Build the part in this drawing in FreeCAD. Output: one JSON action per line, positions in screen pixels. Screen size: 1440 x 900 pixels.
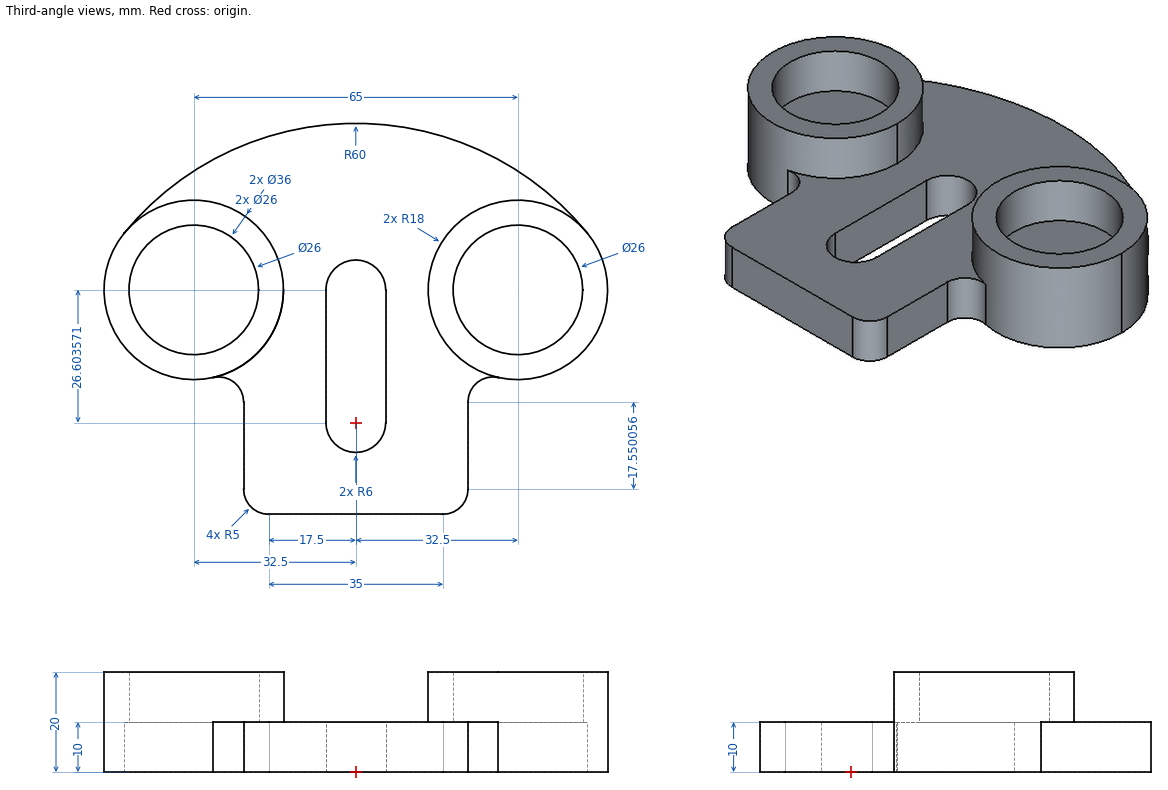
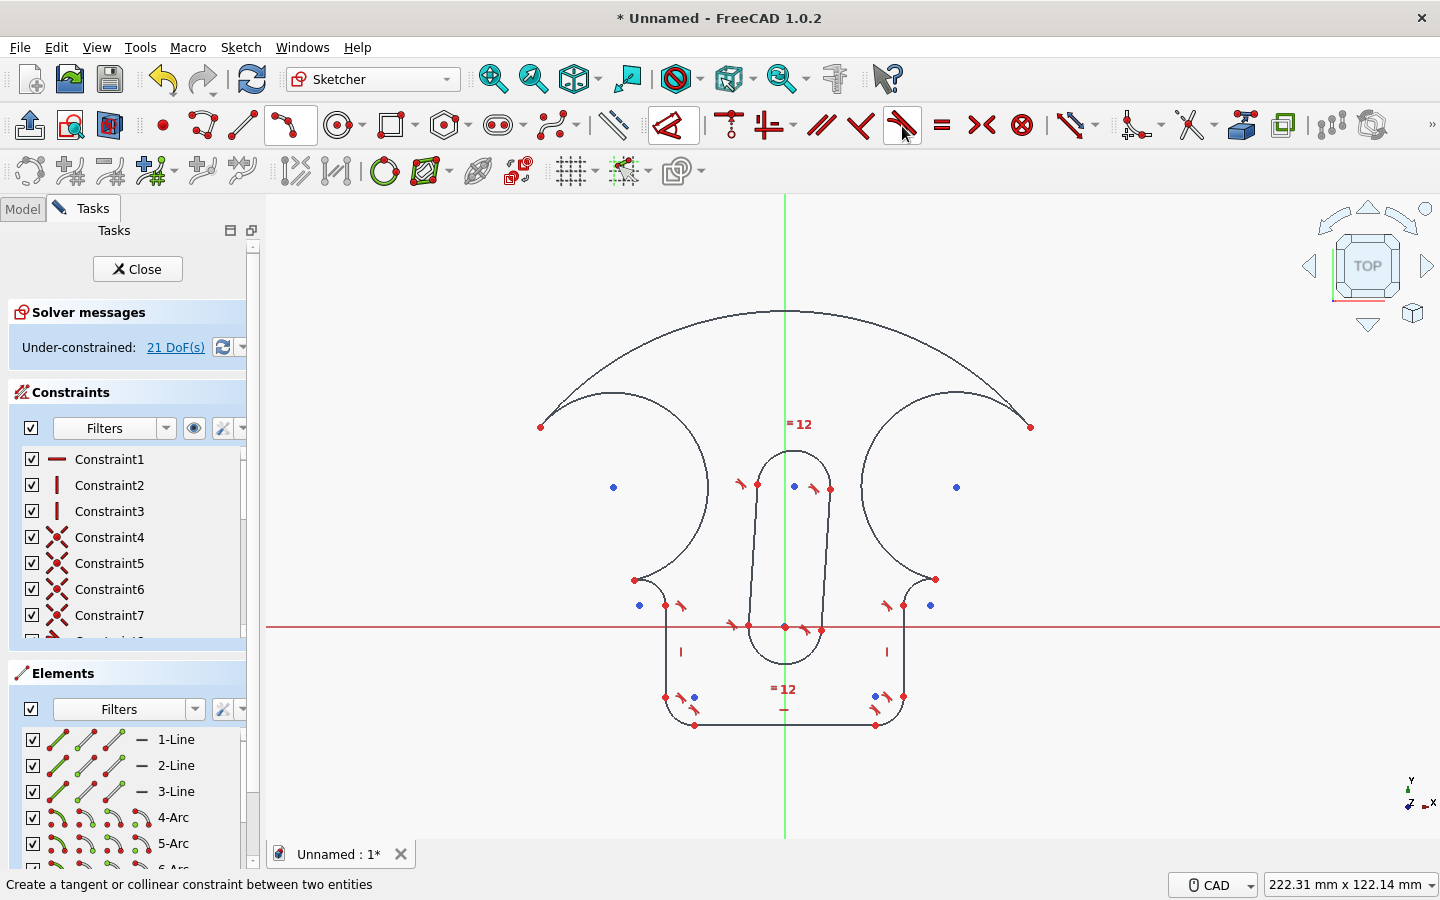
{"action": "left_click", "coordinate": [908, 592]}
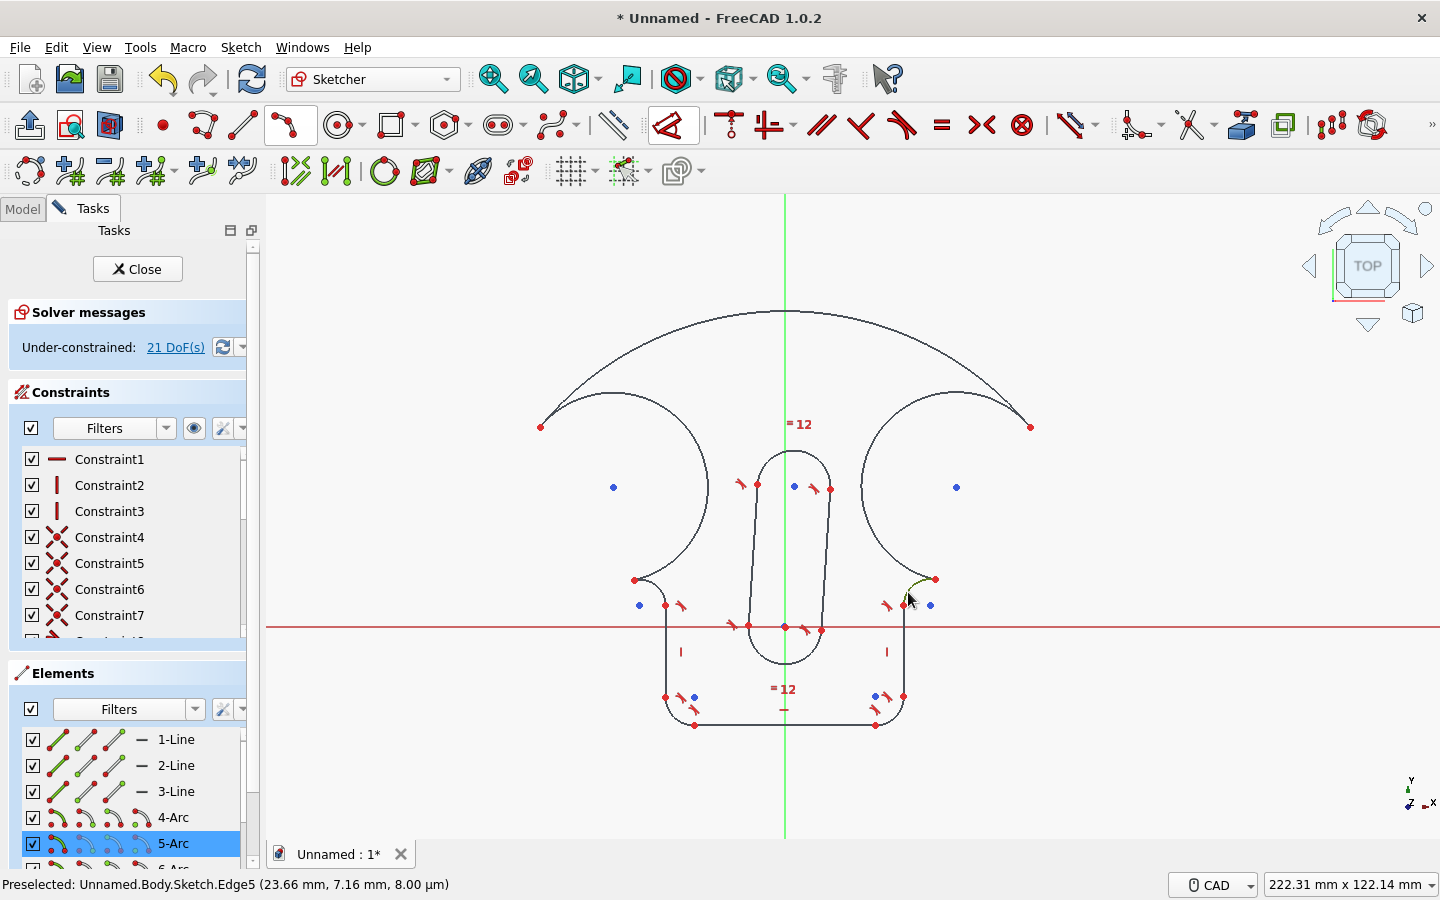
{"action": "left_click", "coordinate": [932, 395]}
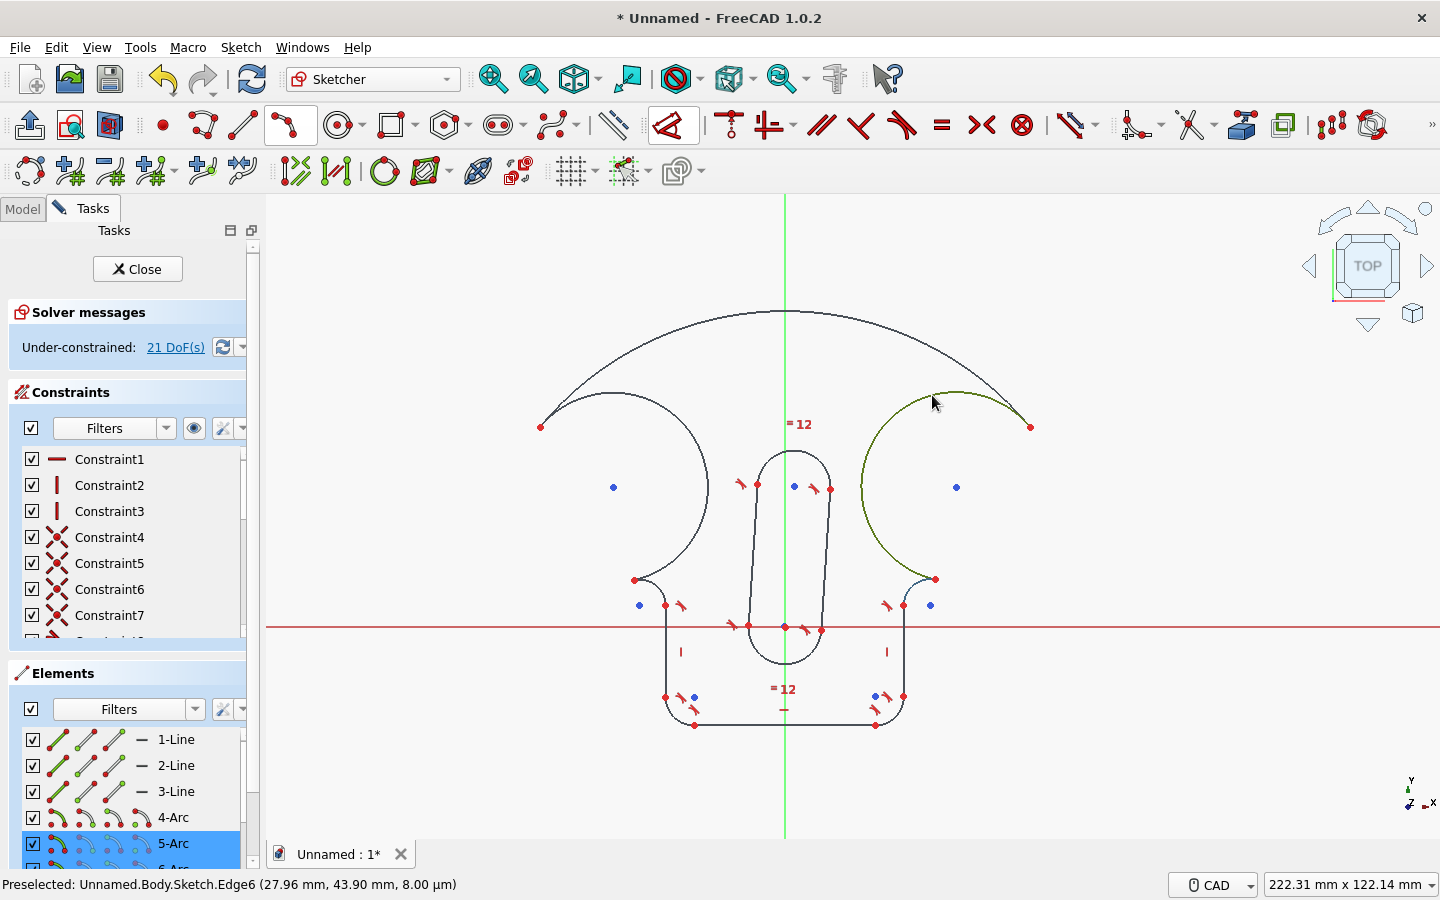
{"action": "left_click", "coordinate": [902, 126]}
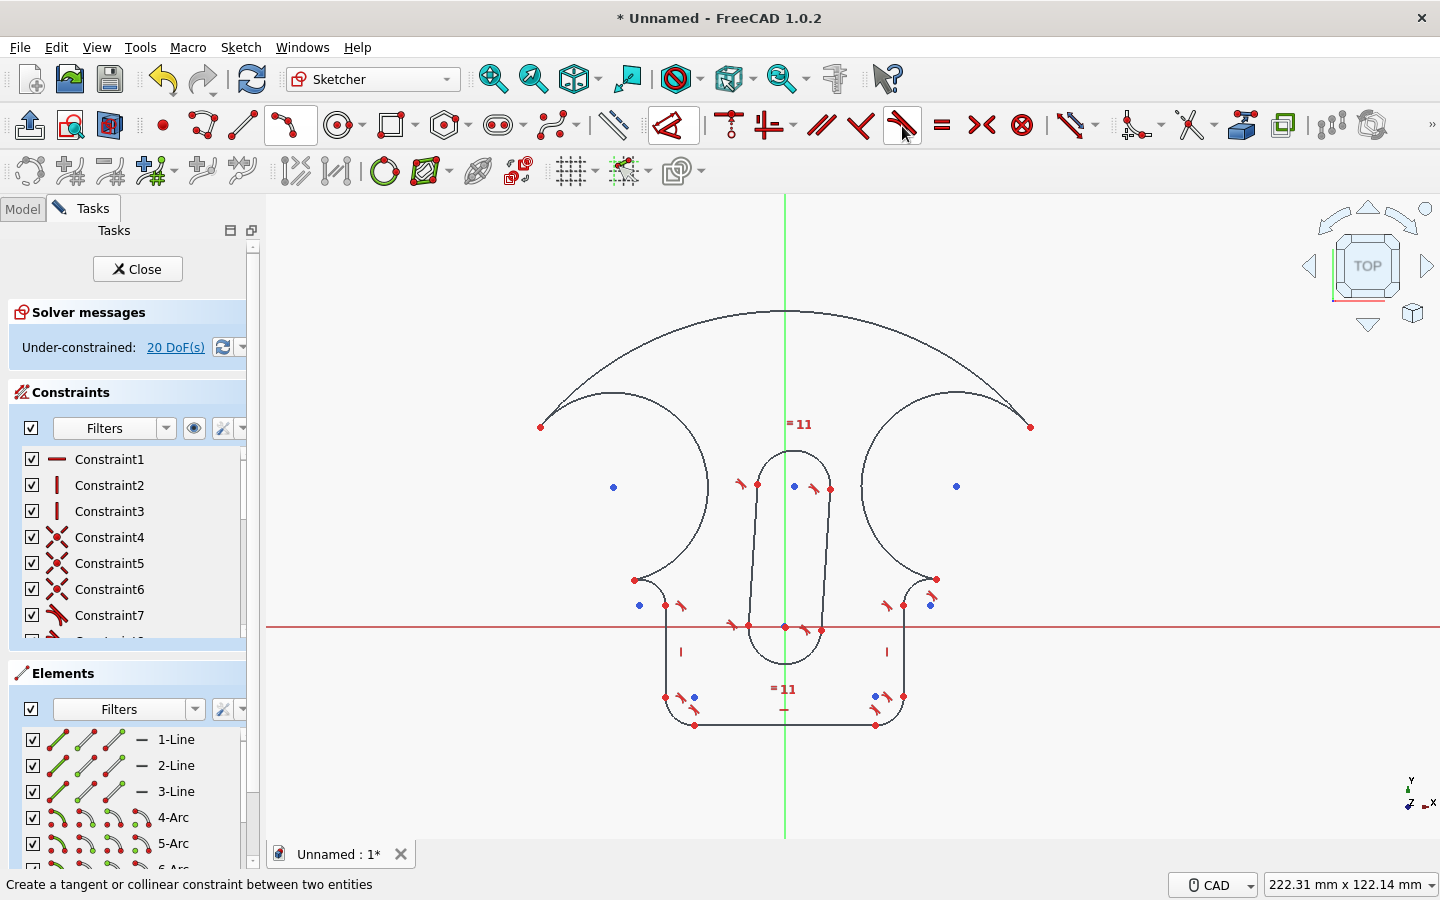
{"action": "left_click", "coordinate": [932, 395]}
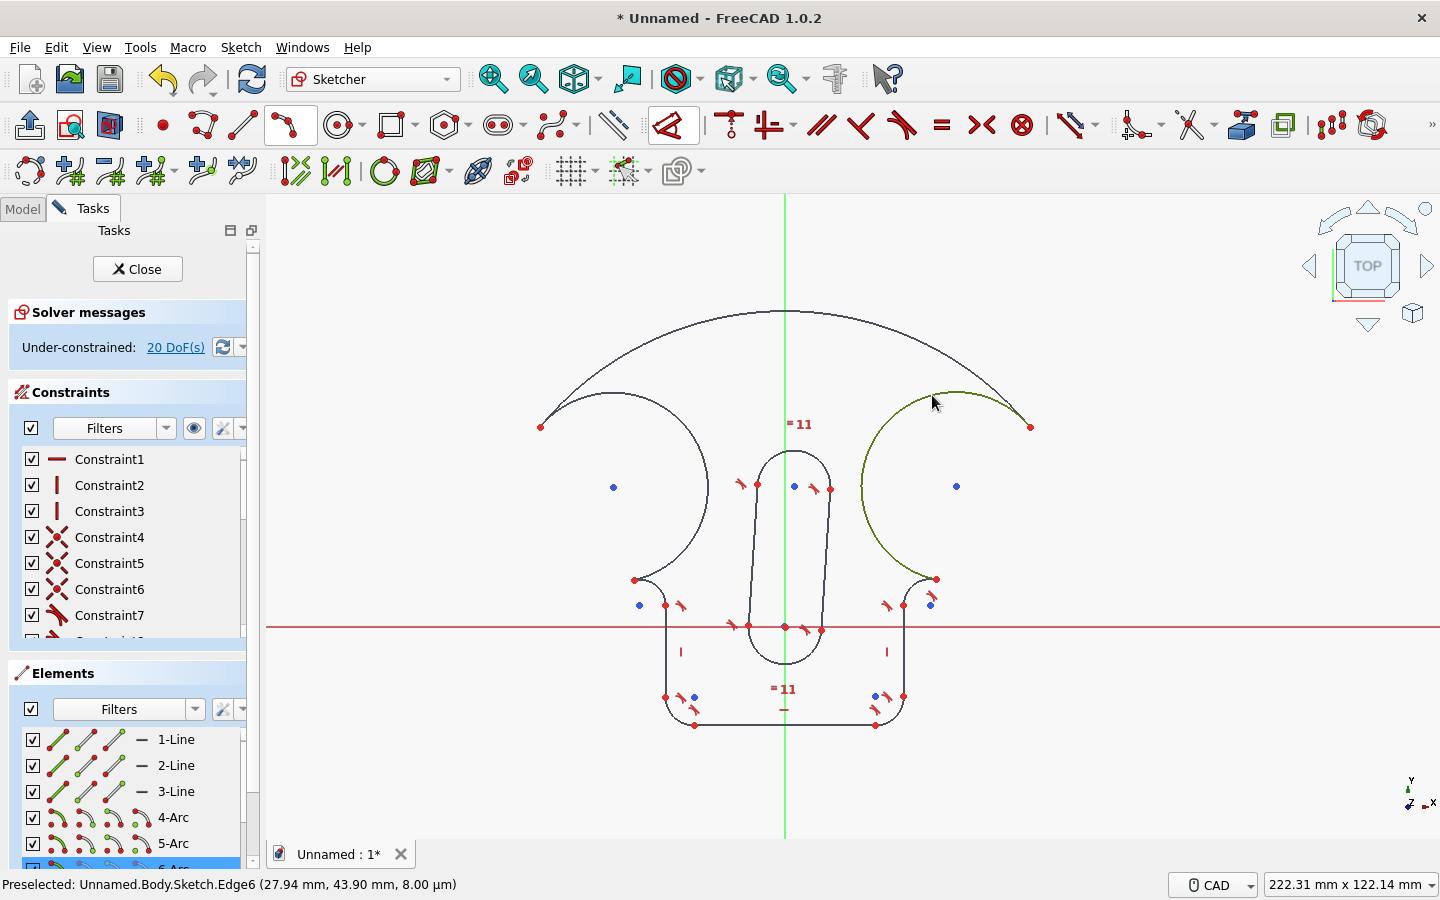
{"action": "left_click", "coordinate": [895, 331]}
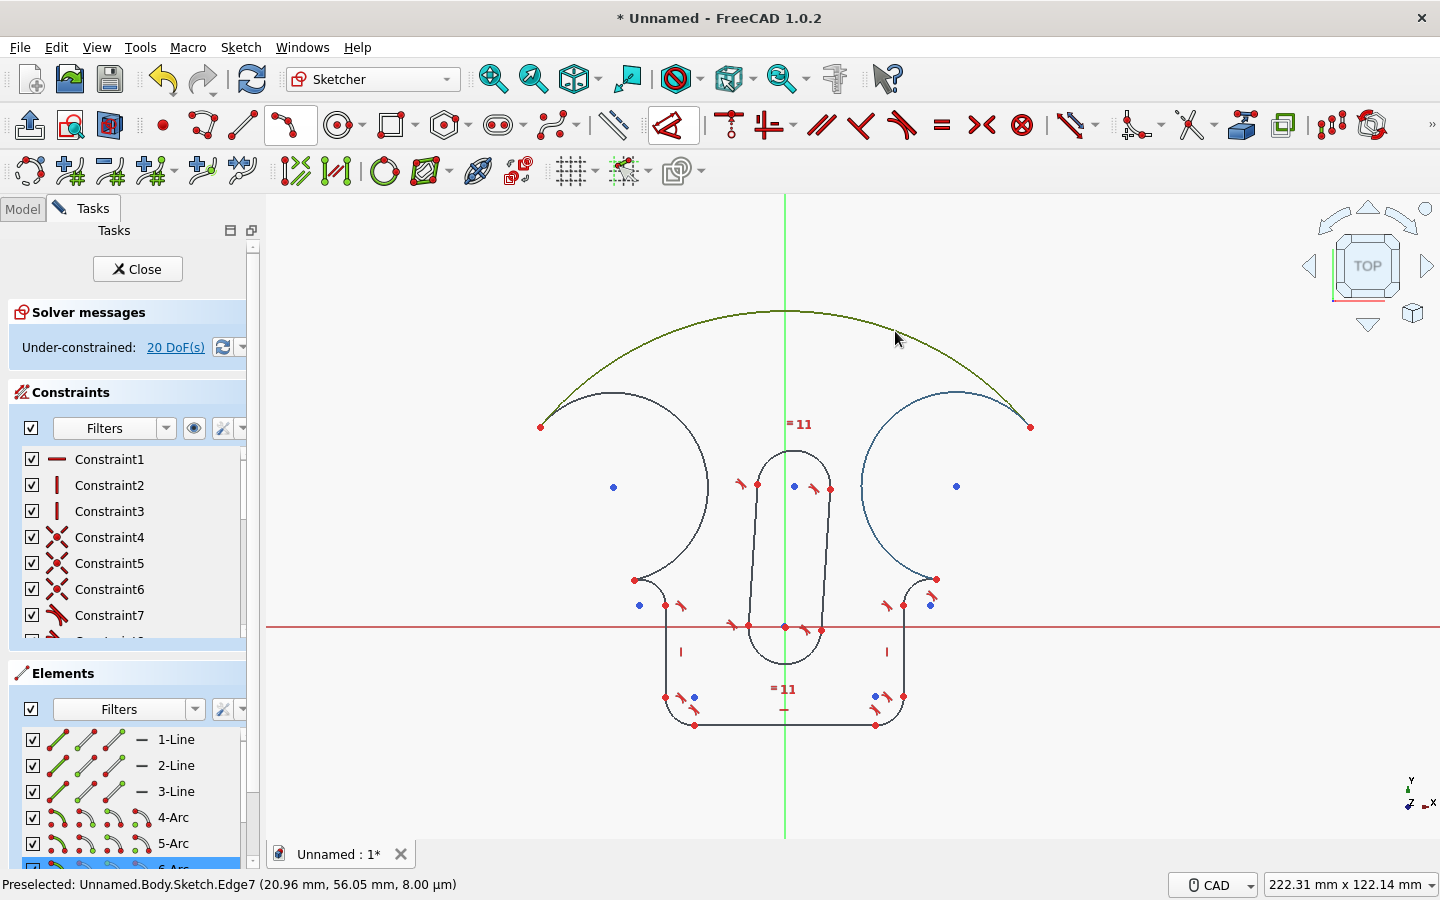
{"action": "left_click", "coordinate": [902, 126]}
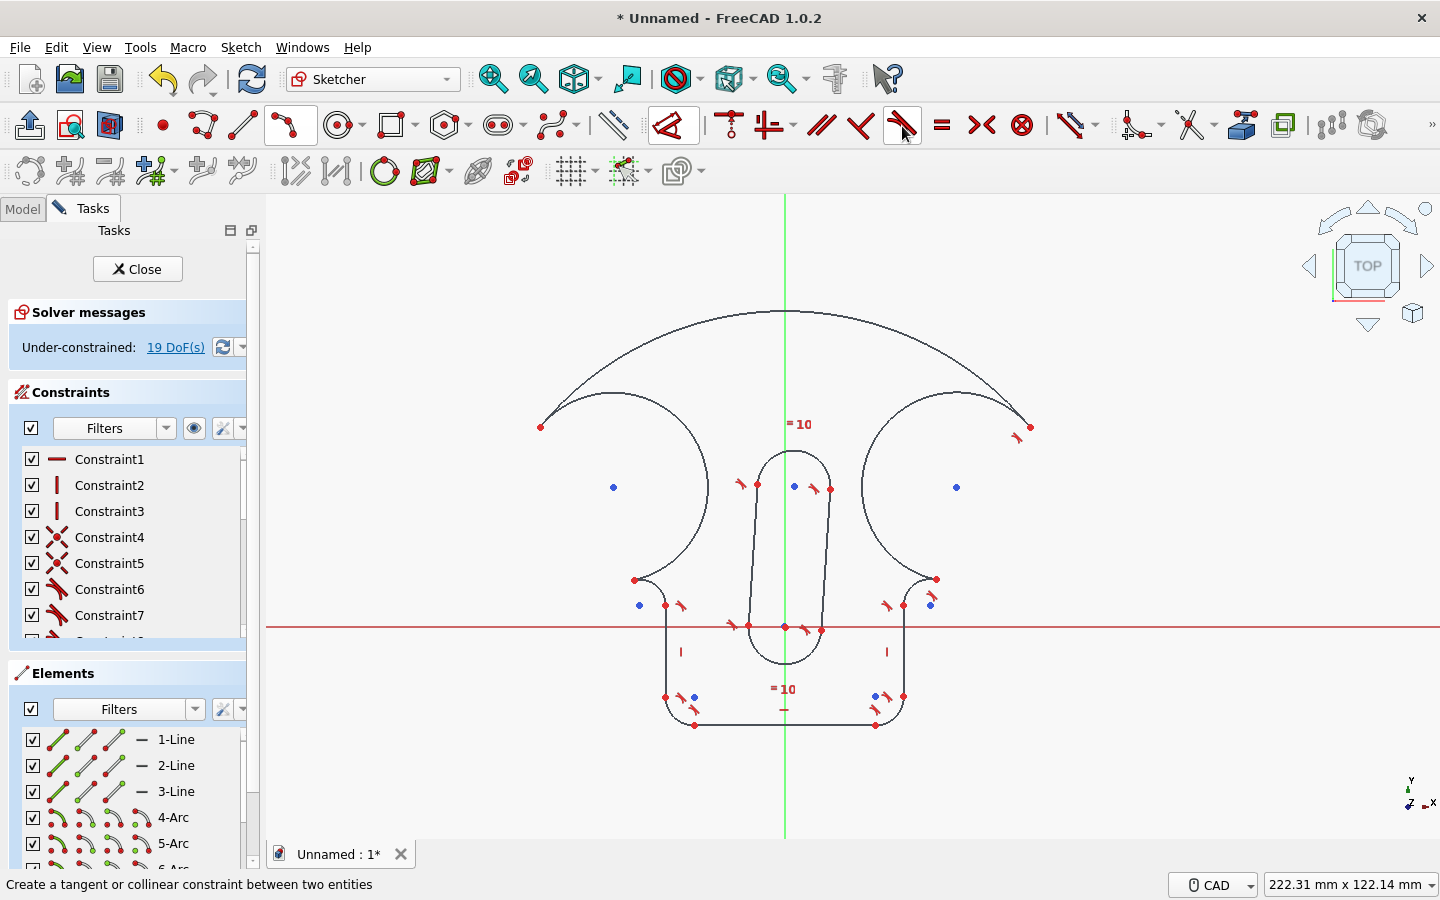
{"action": "left_click", "coordinate": [895, 331]}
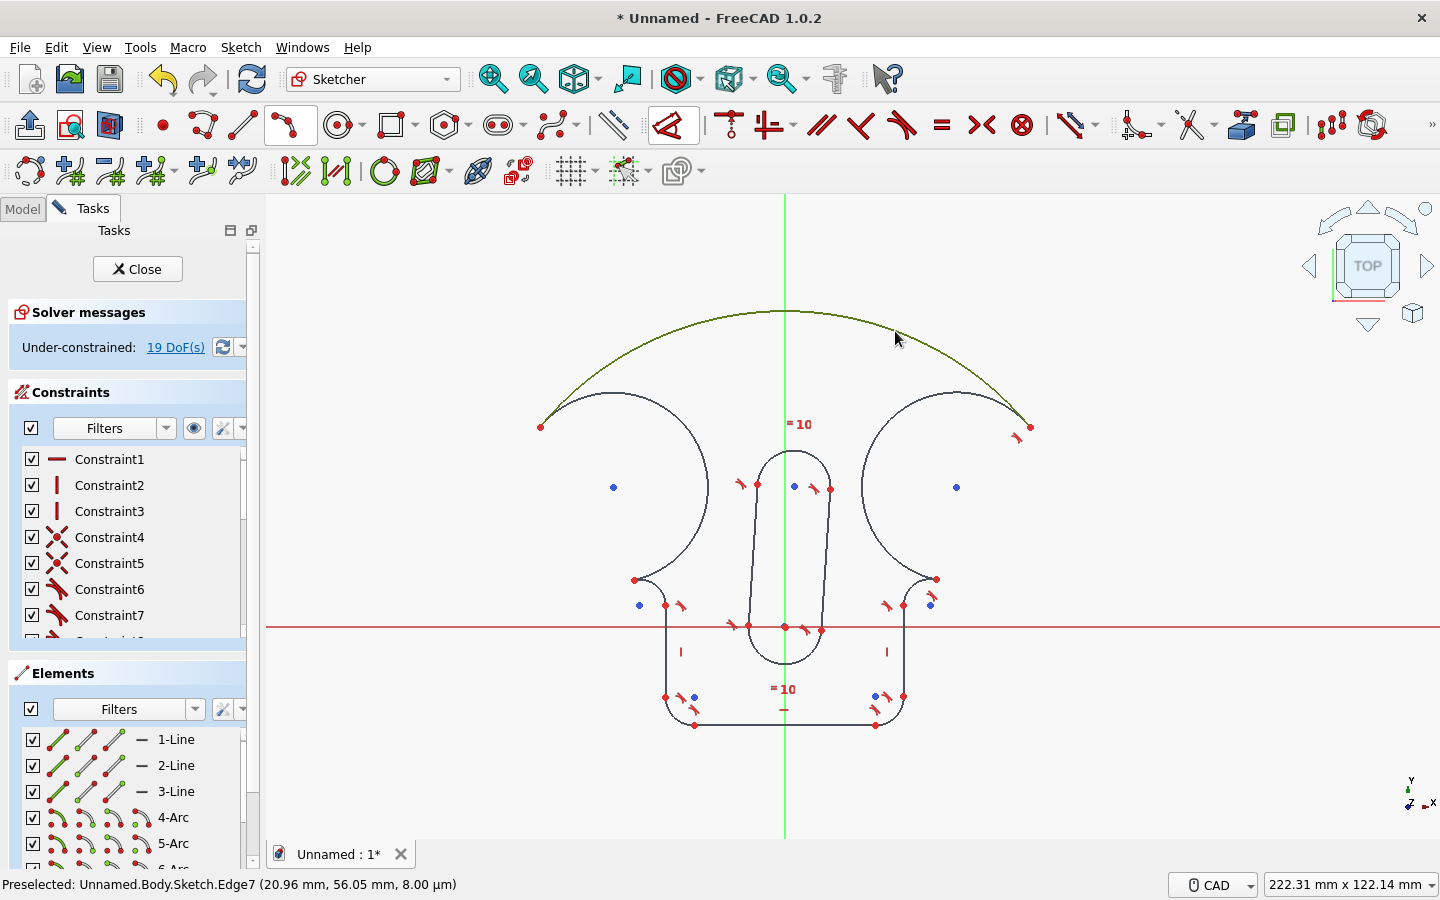
{"action": "left_click", "coordinate": [706, 507]}